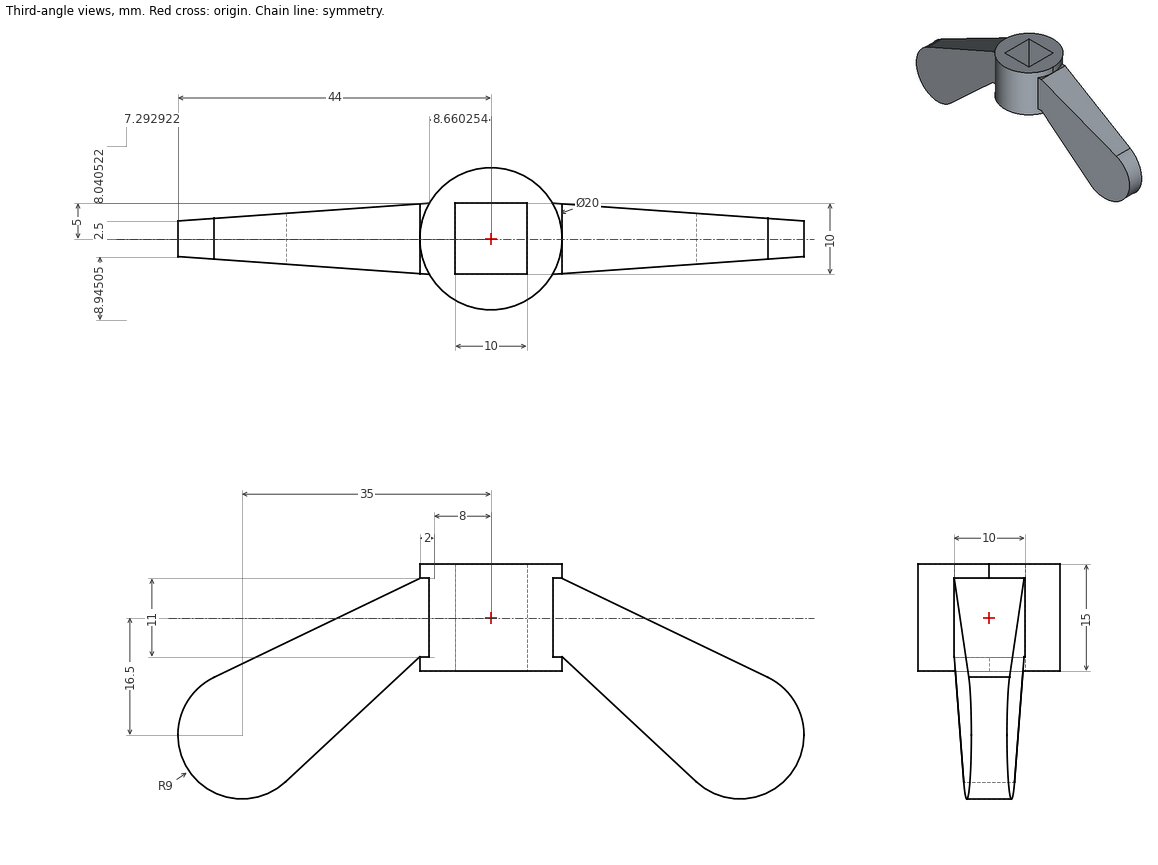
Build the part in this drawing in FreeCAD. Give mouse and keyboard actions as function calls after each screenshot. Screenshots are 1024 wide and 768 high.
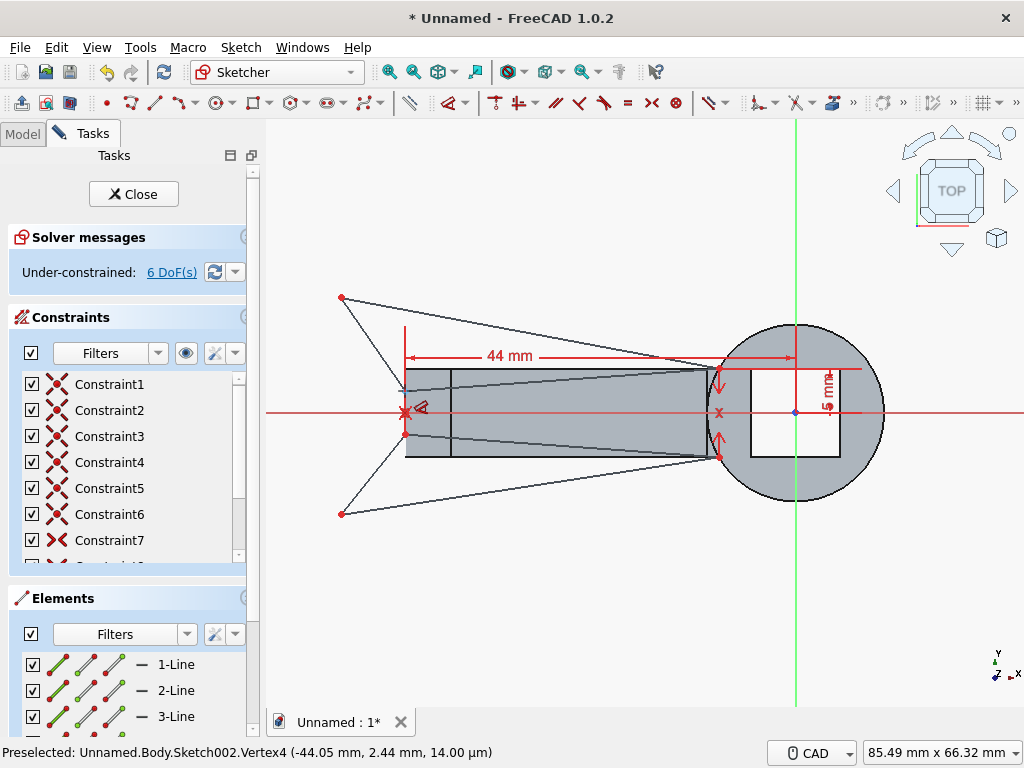
click(406, 391)
click(372, 411)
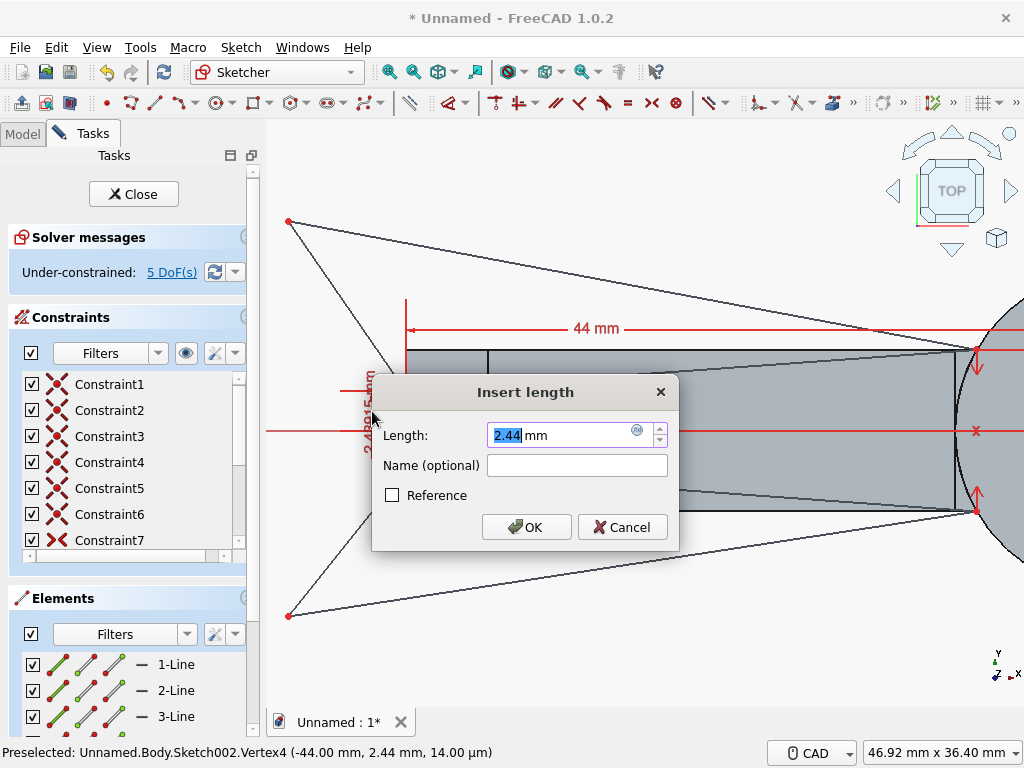
text(2.5)
key(Return)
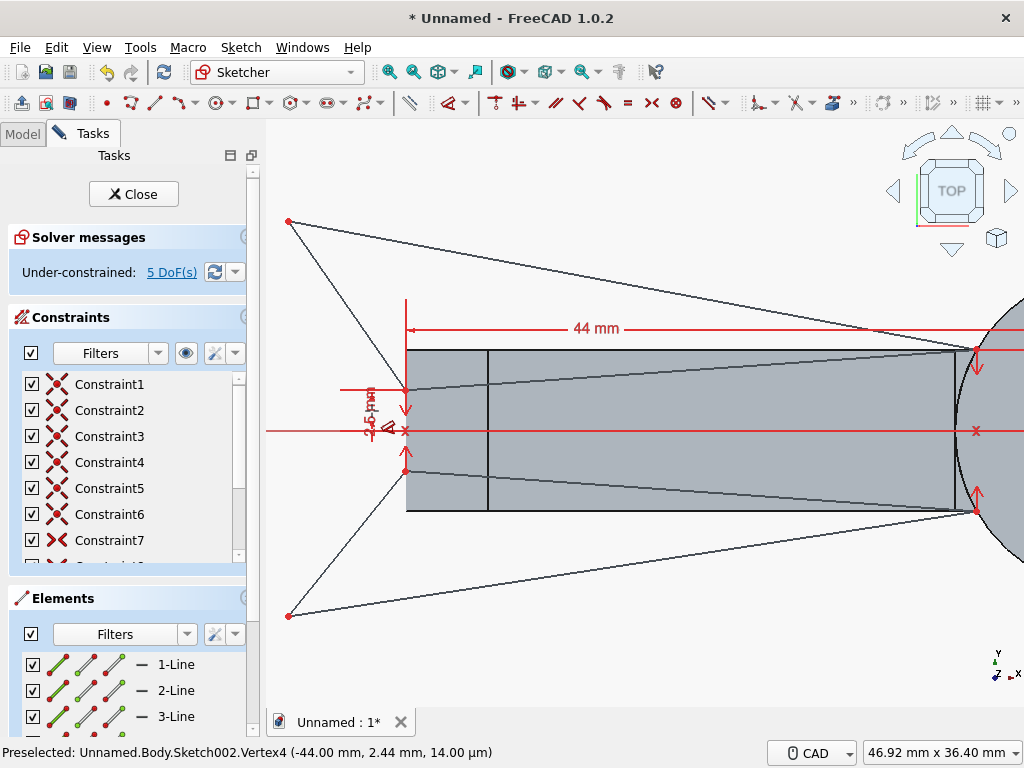
click(370, 515)
click(440, 544)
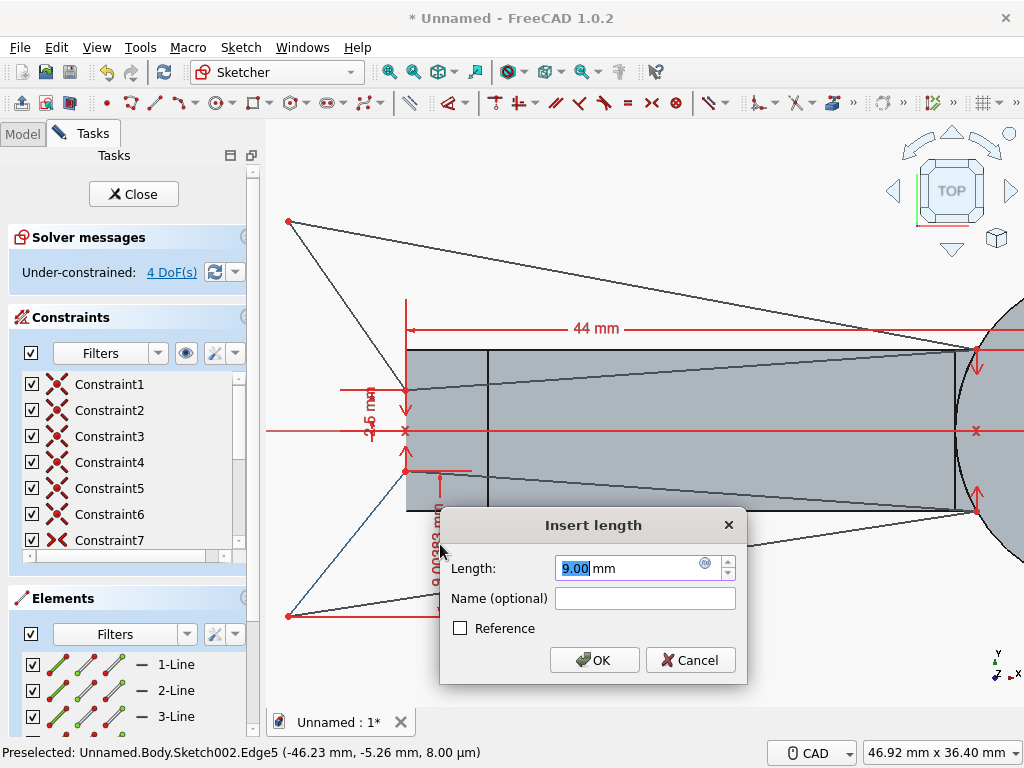
text(8.94505)
key(Return)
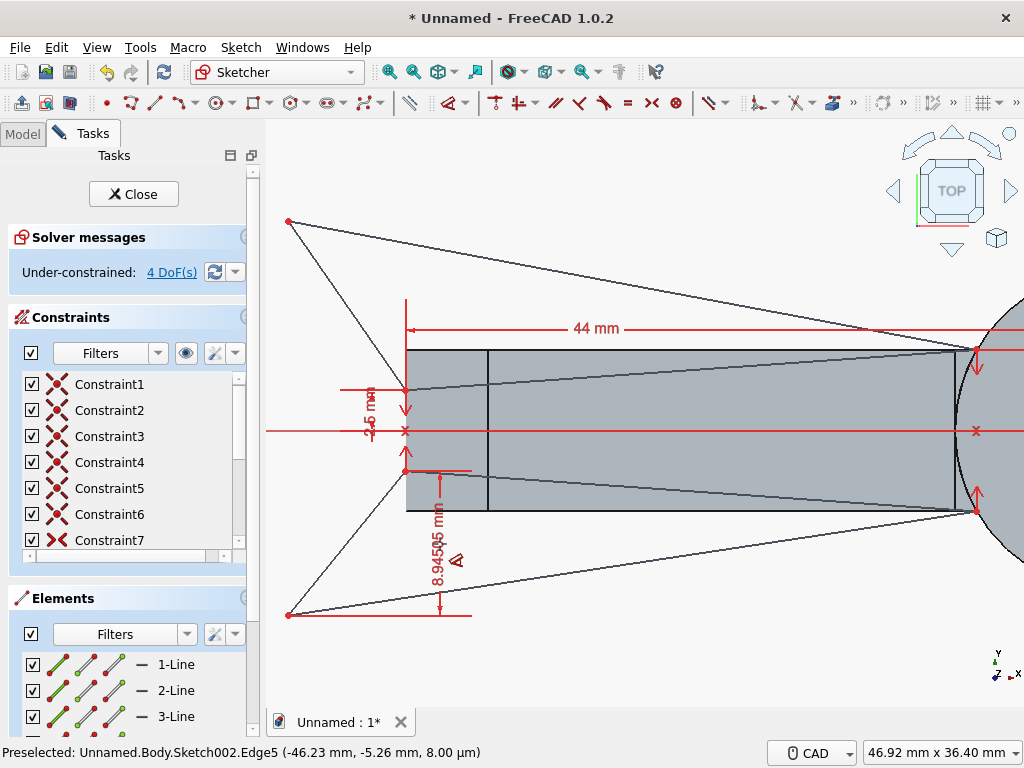
scroll(474, 409, down, 4)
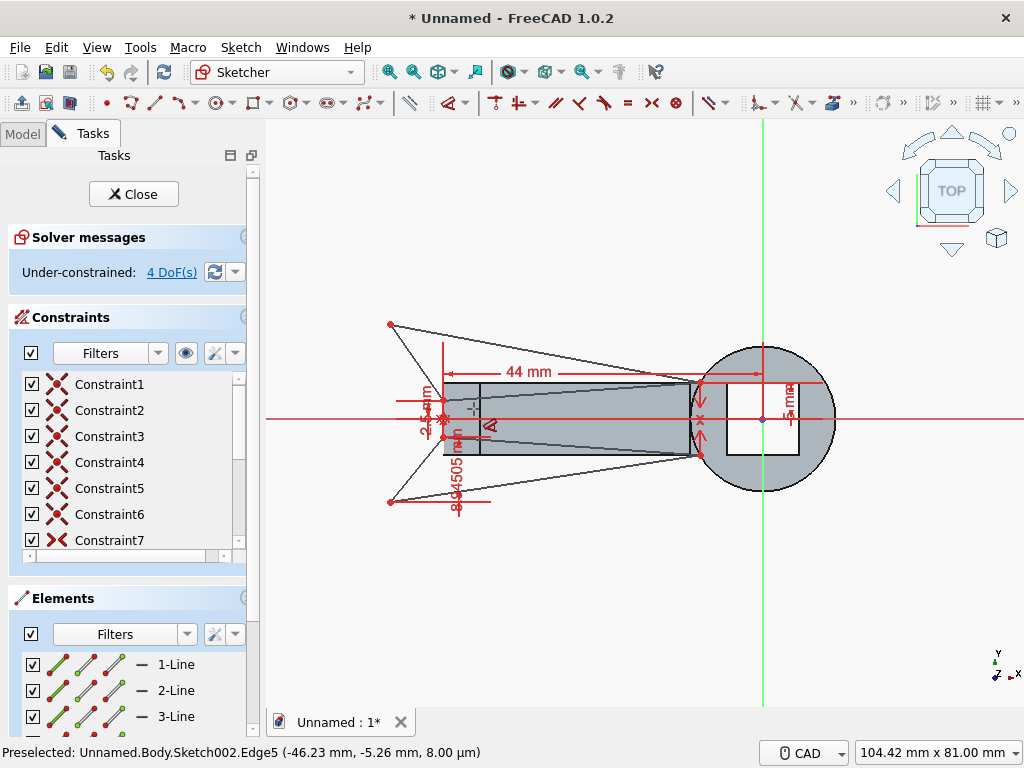
click(700, 383)
click(732, 349)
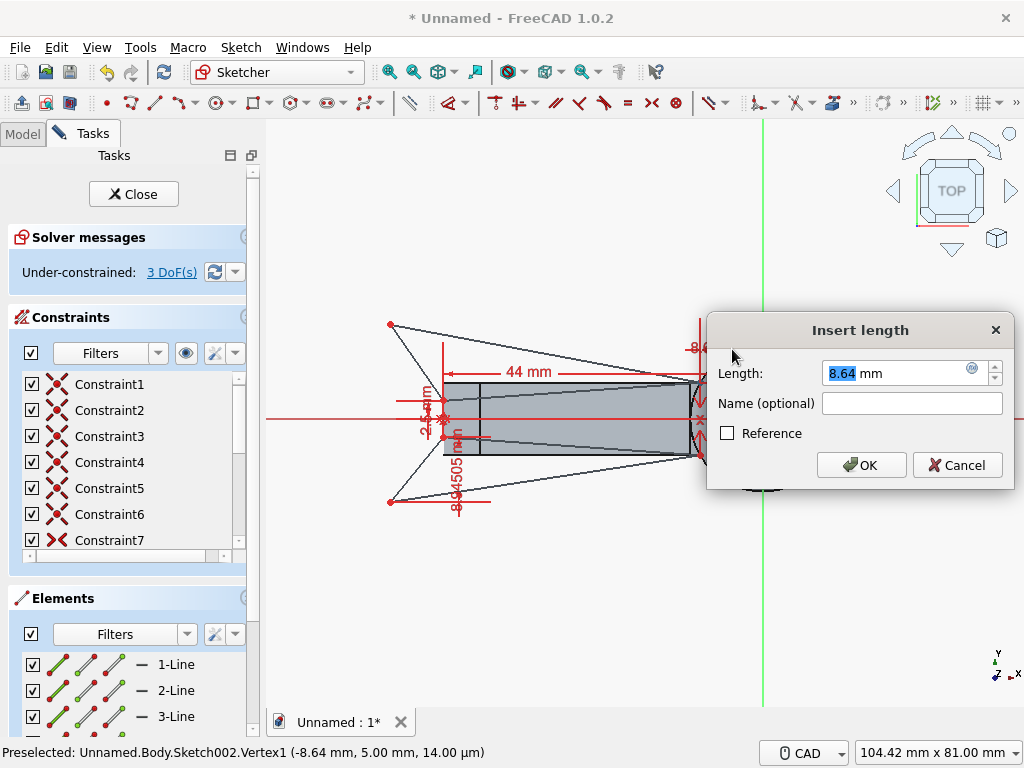
text(8.660254)
key(Return)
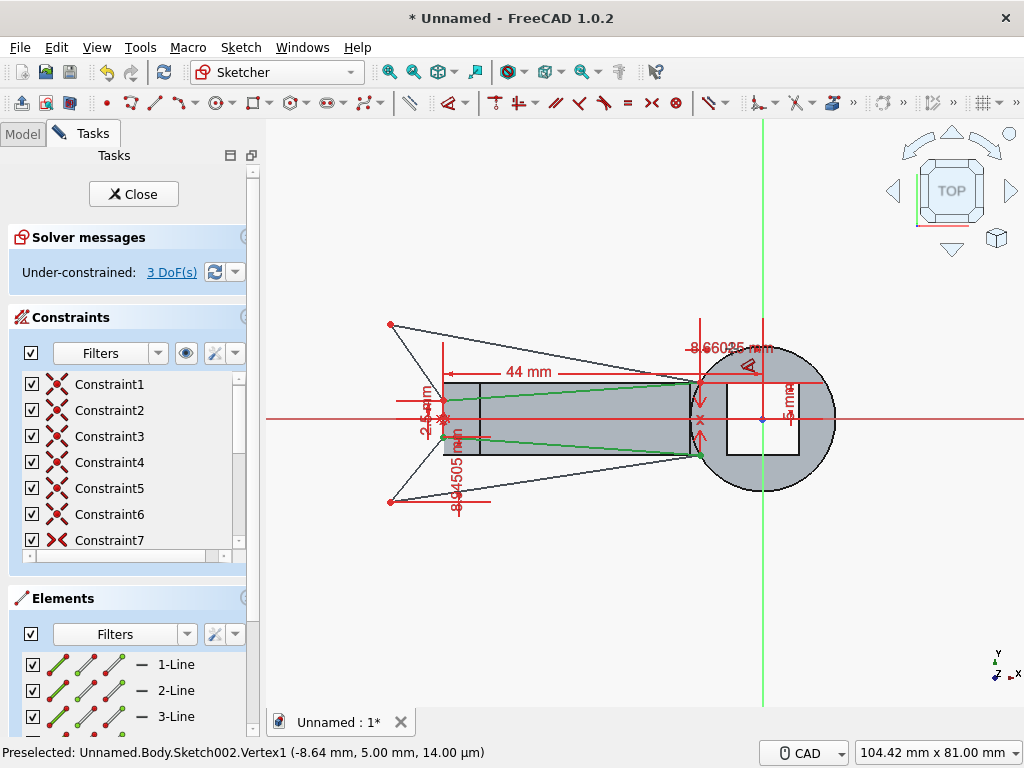
click(607, 365)
click(357, 354)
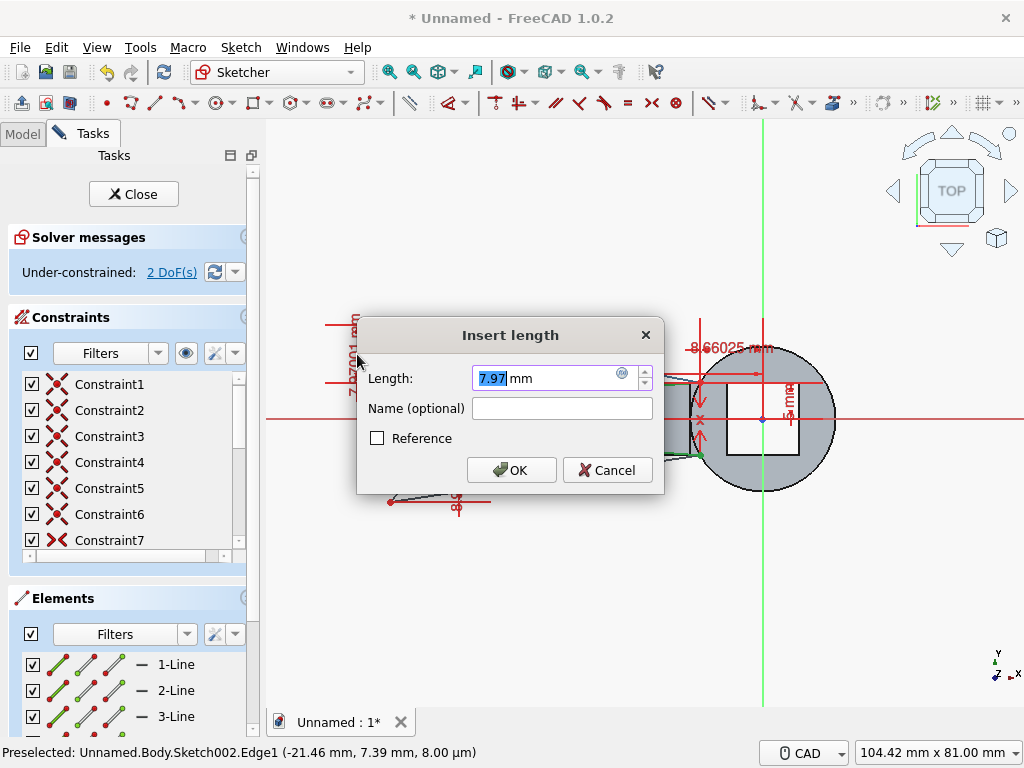
text(8.040522)
key(Return)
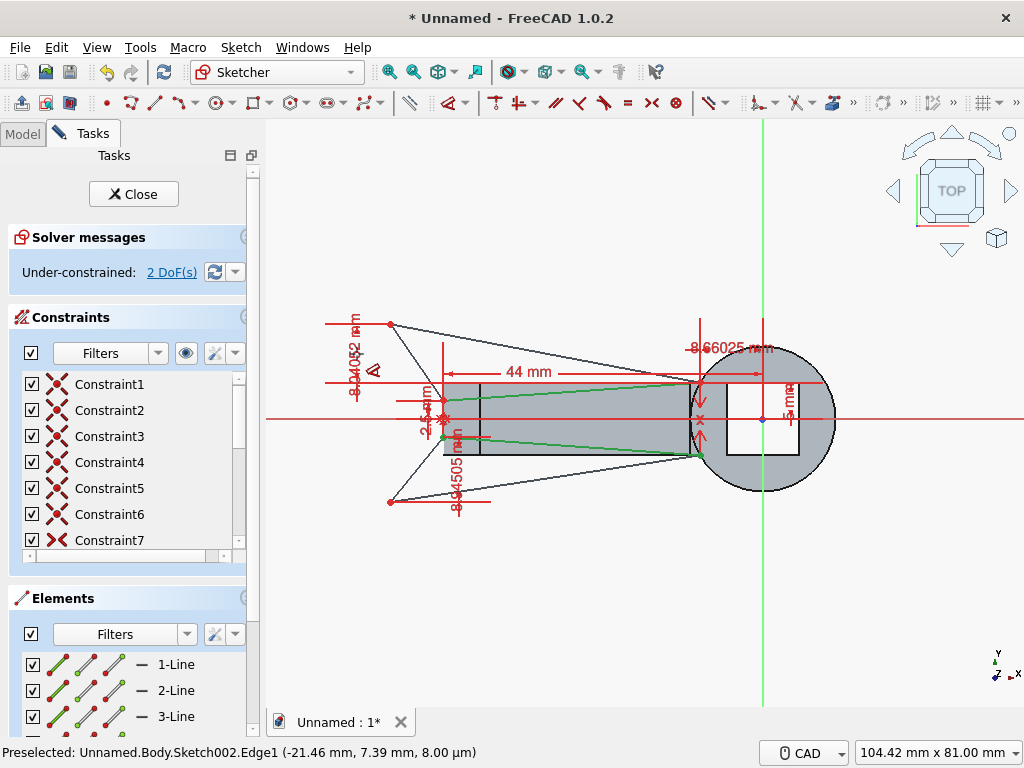
click(407, 347)
click(417, 290)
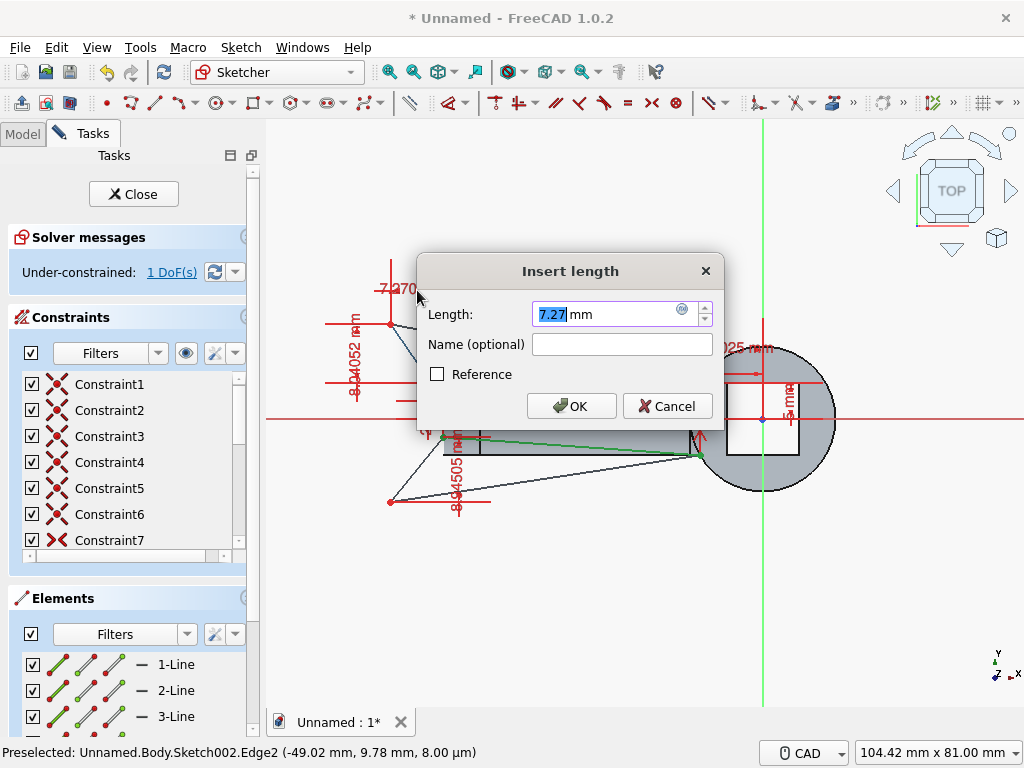
text(7.292922)
key(Return)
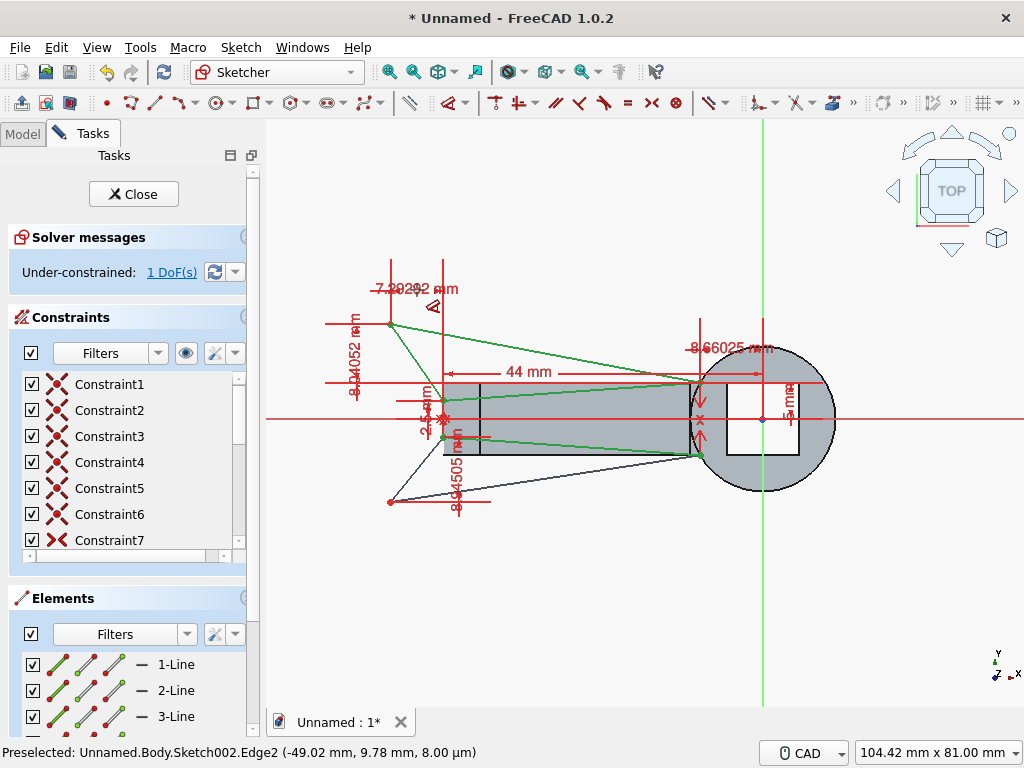
click(428, 457)
click(417, 536)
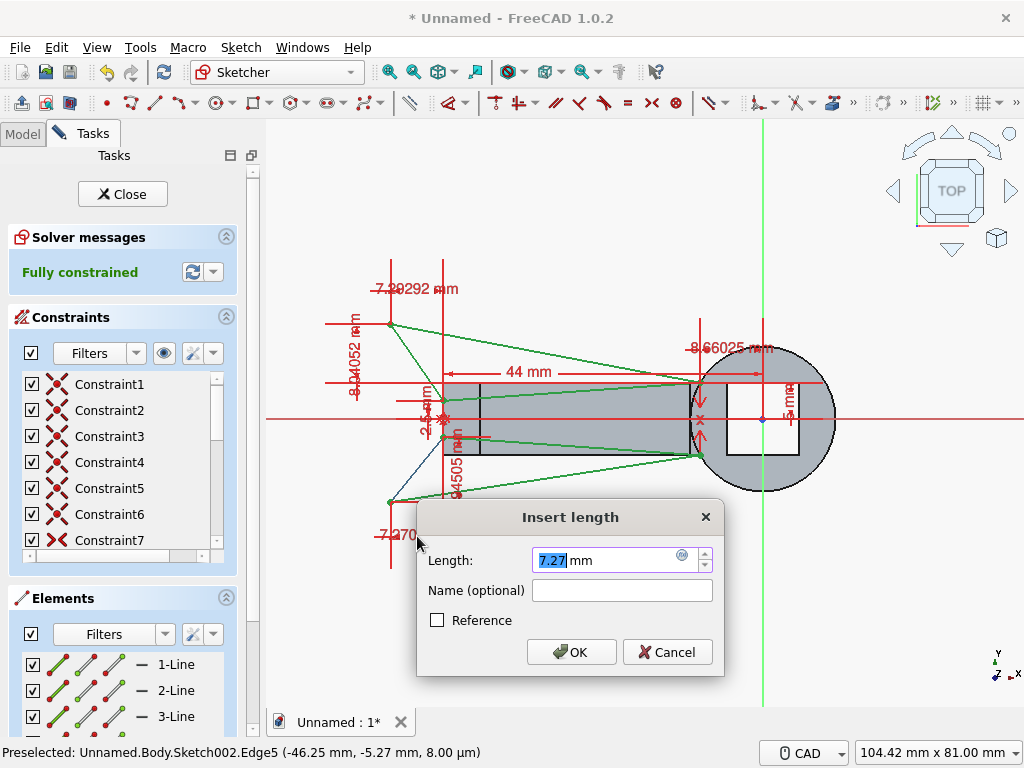
text(7.292922)
key(Return)
key(Escape)